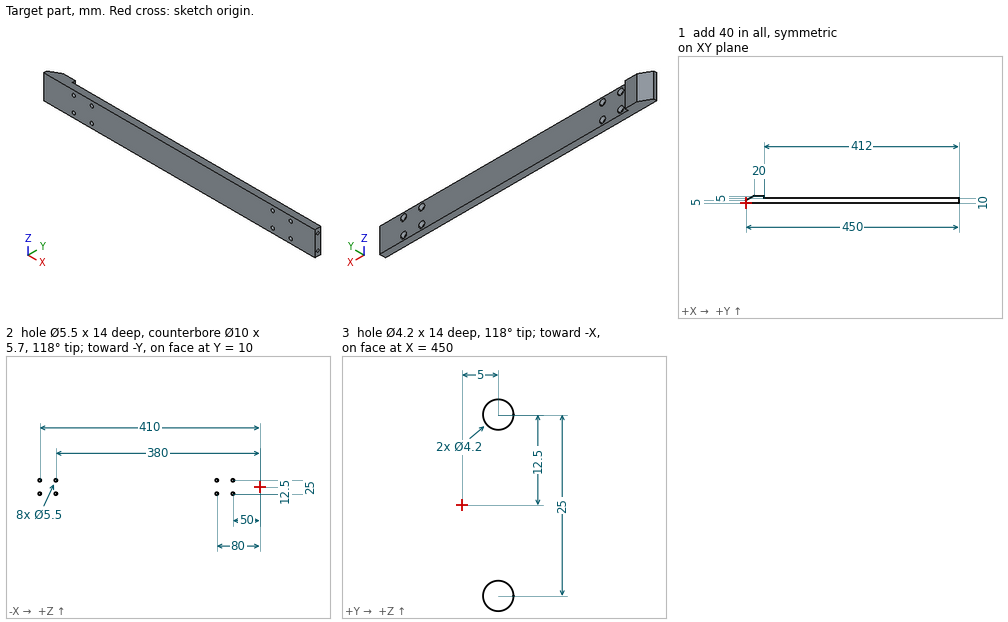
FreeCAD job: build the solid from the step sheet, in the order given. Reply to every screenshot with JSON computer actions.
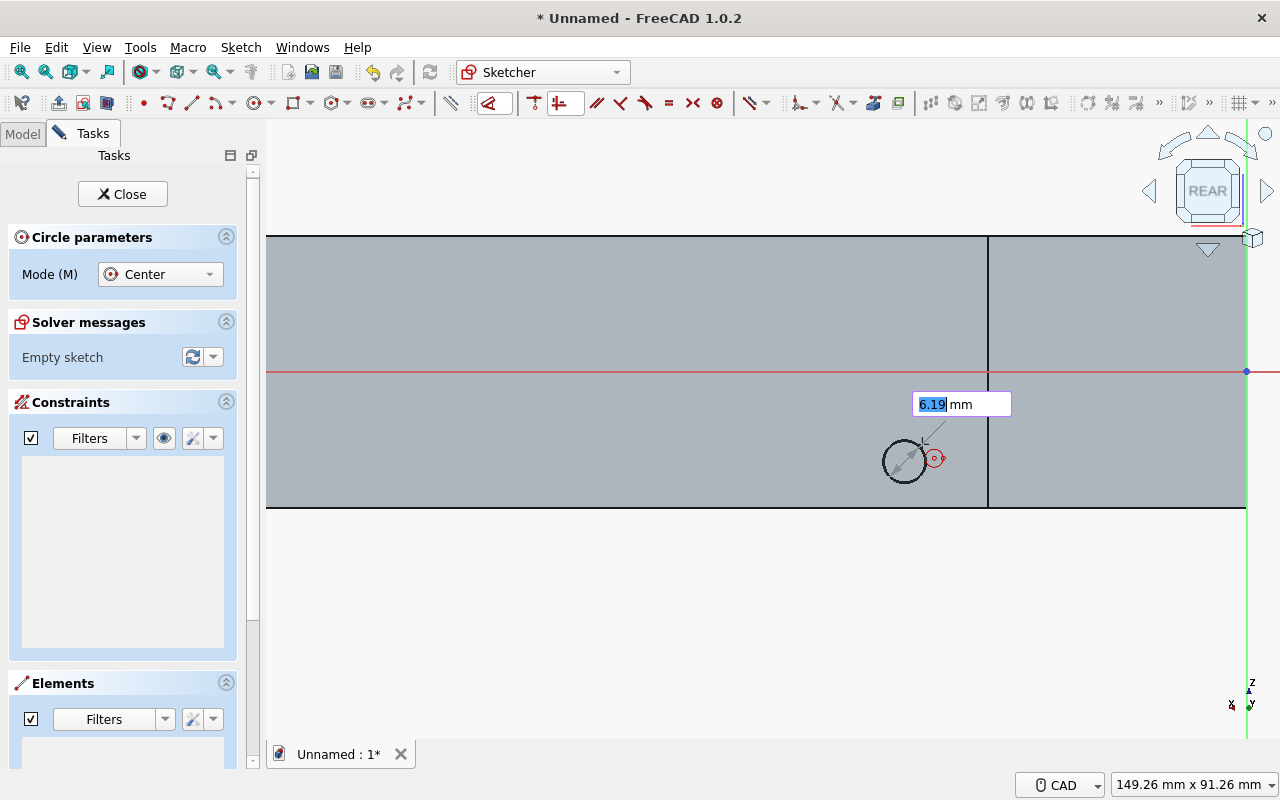
{"action": "left_click", "coordinate": [920, 443]}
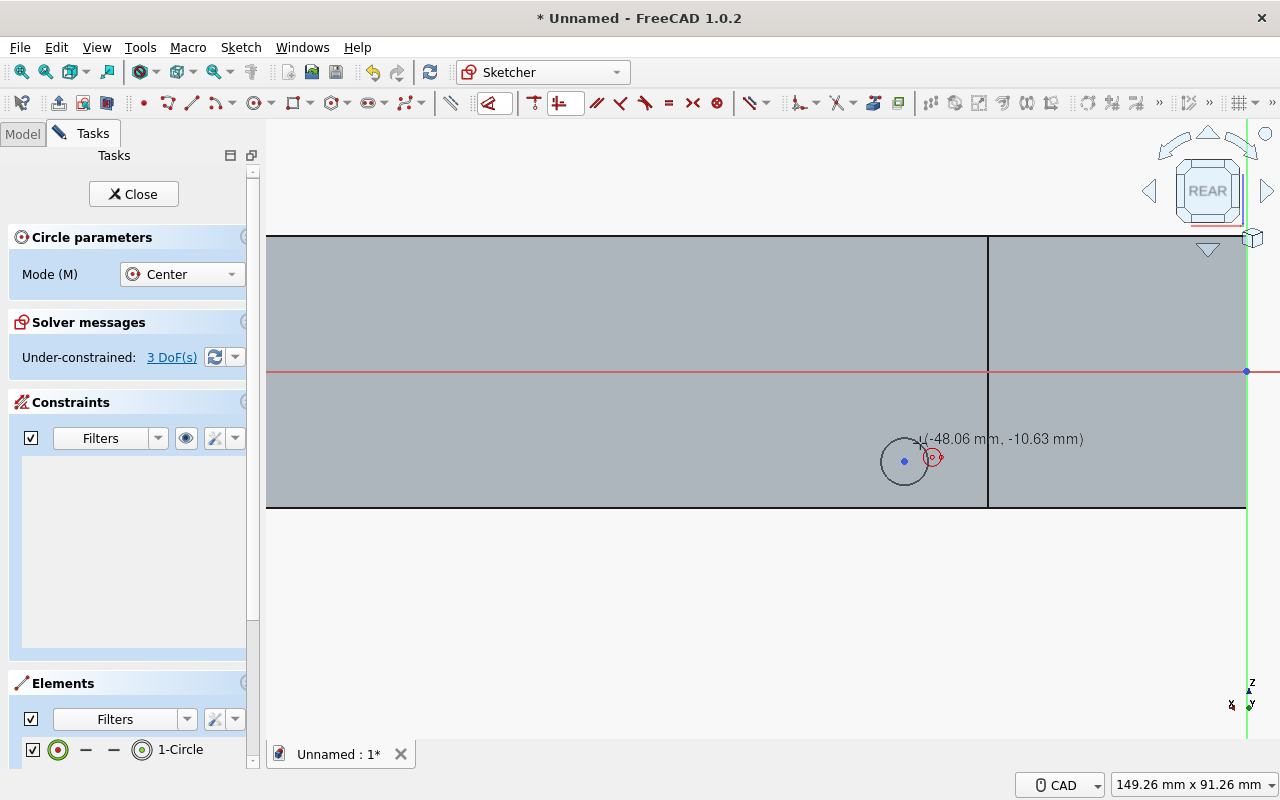
{"action": "scroll", "coordinate": [922, 443], "scroll_direction": "down", "scroll_amount": 8}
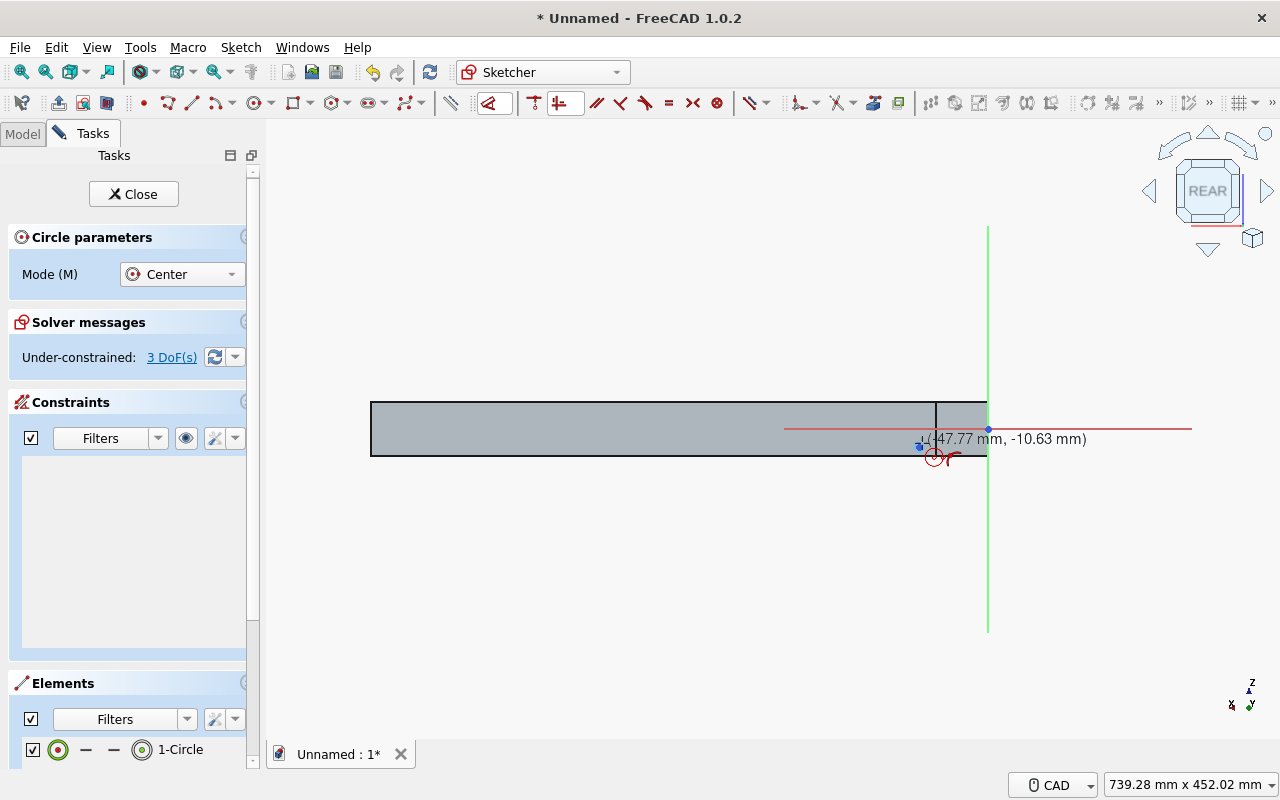
{"action": "left_click", "coordinate": [878, 446]}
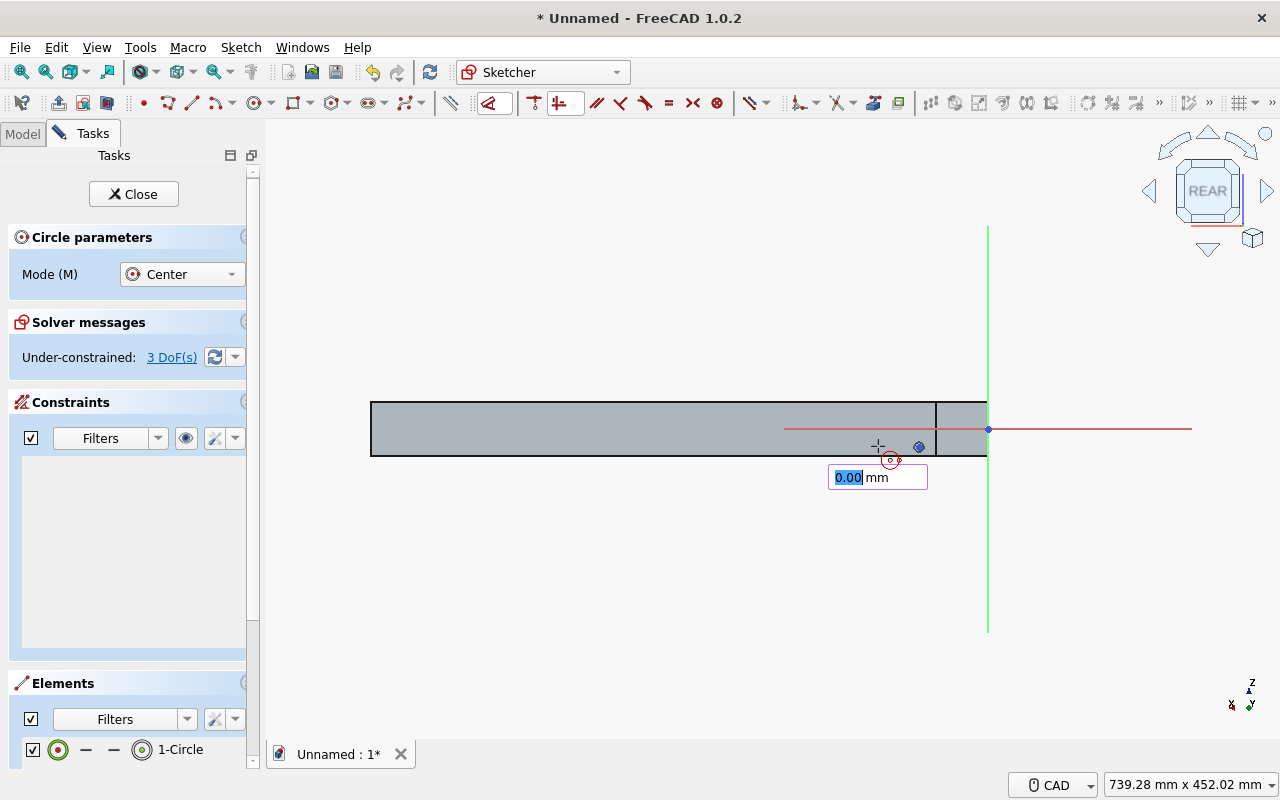
{"action": "scroll", "coordinate": [881, 444], "scroll_direction": "up", "scroll_amount": 8}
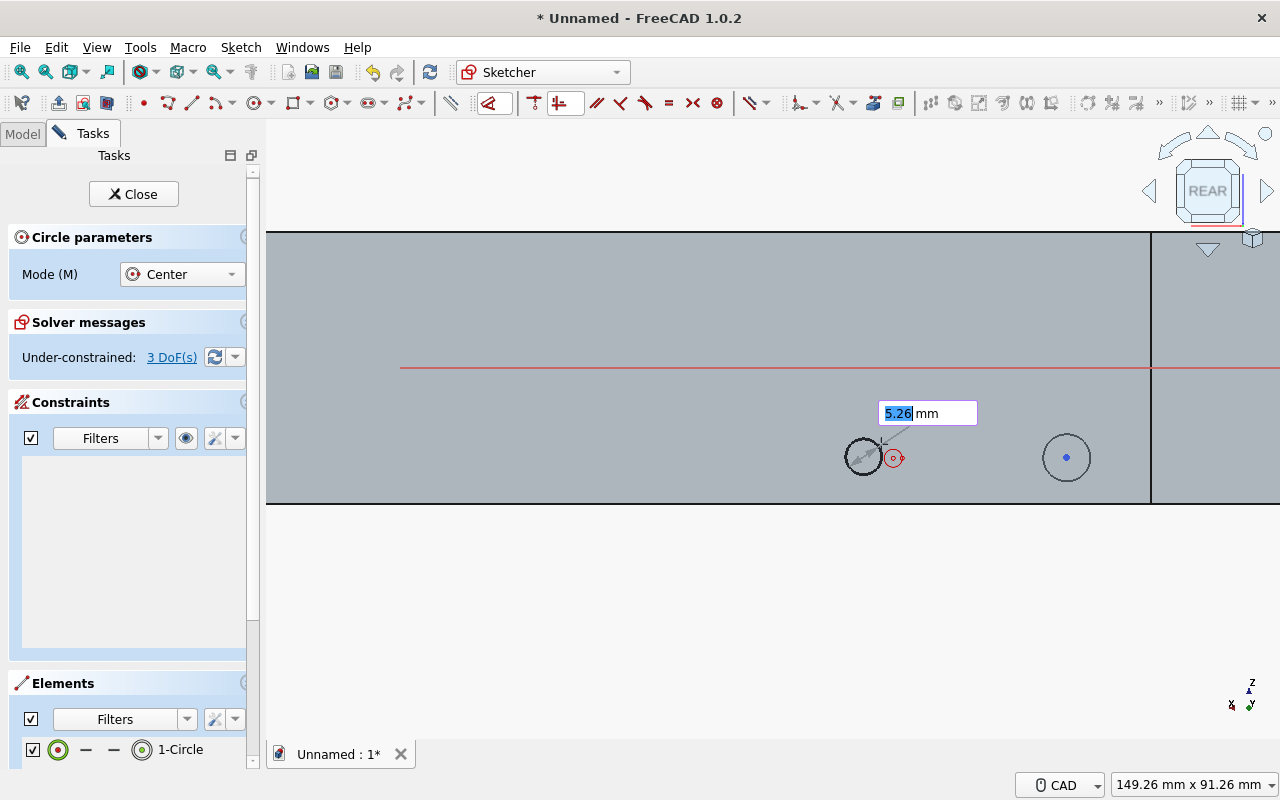
{"action": "left_click", "coordinate": [878, 440]}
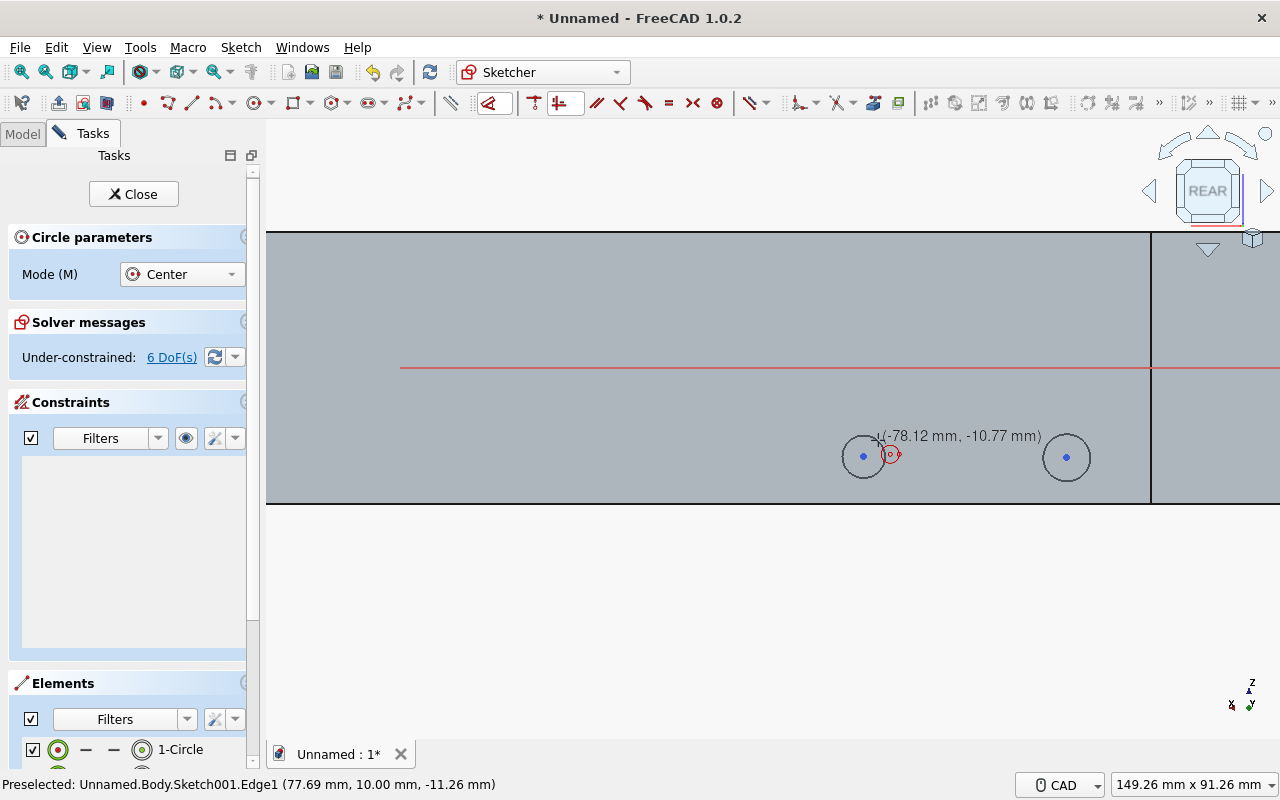
{"action": "scroll", "coordinate": [881, 444], "scroll_direction": "down", "scroll_amount": 8}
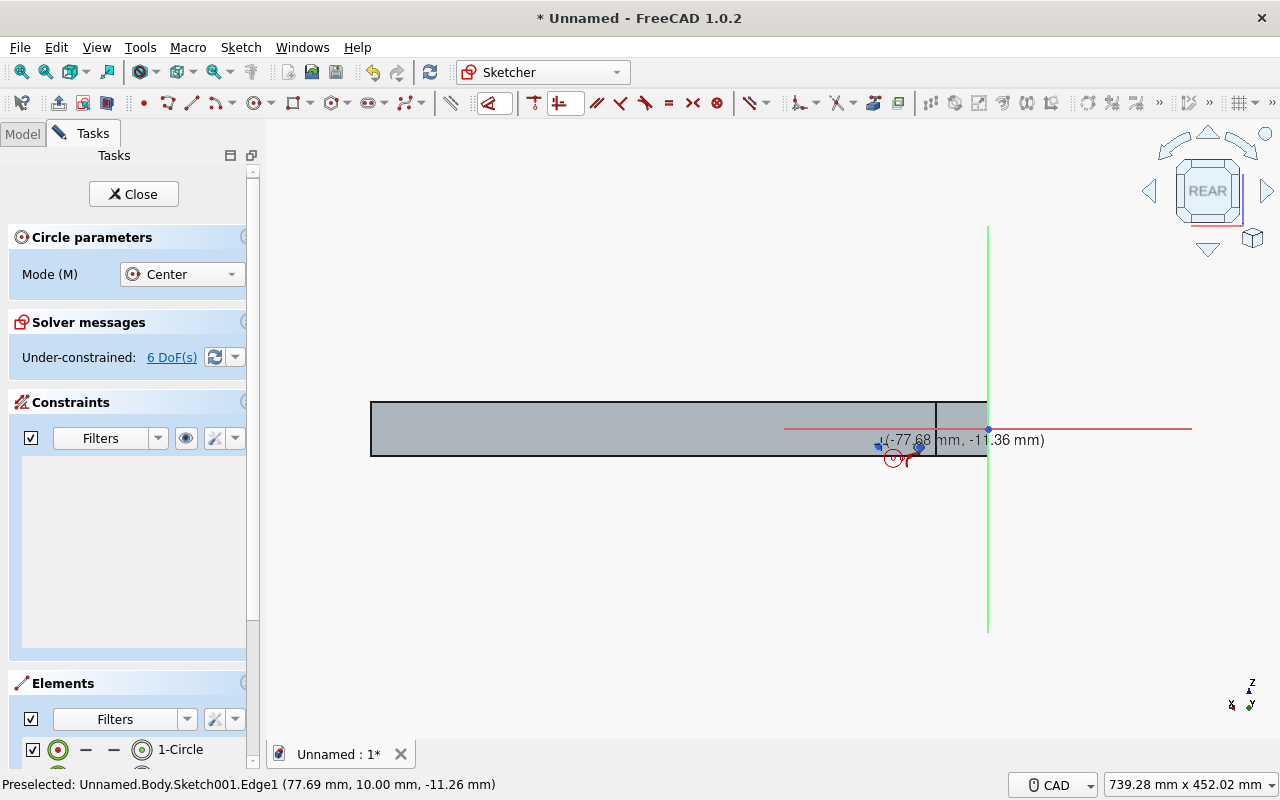
{"action": "left_click", "coordinate": [919, 412]}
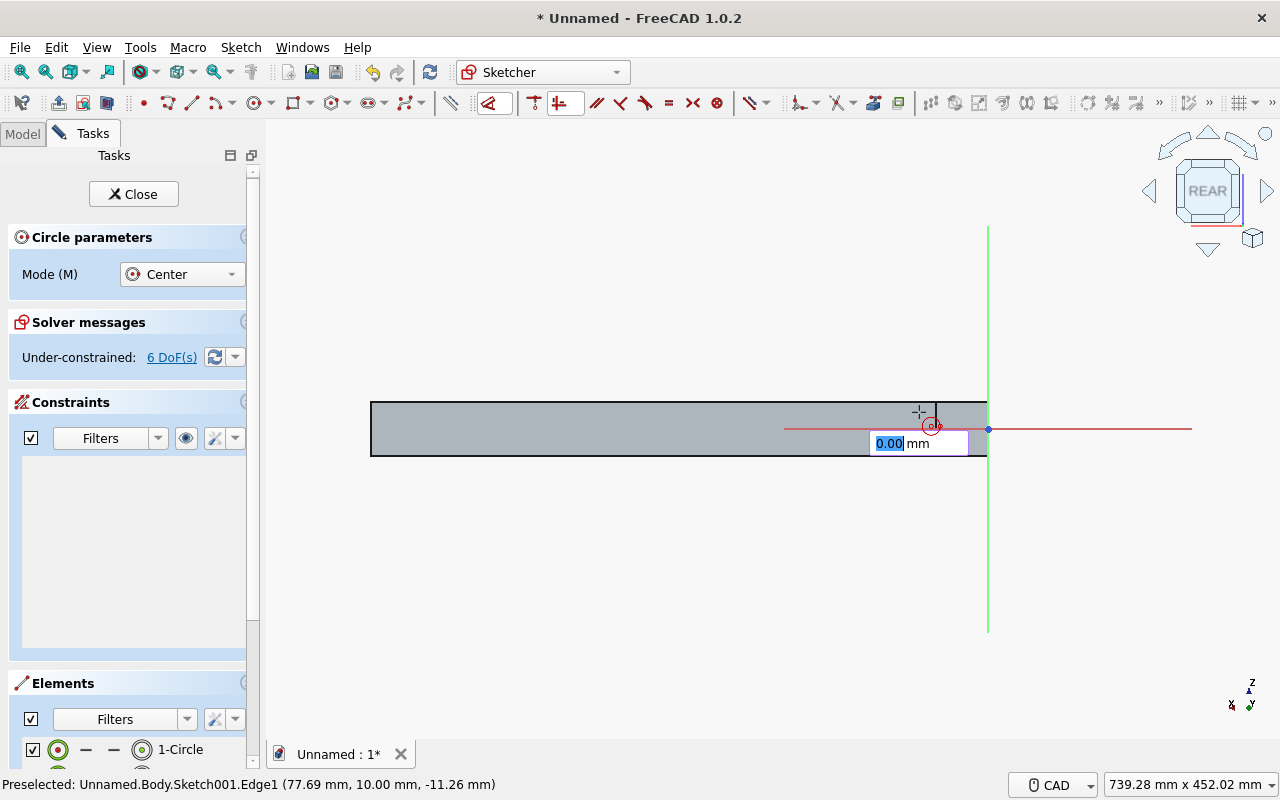
{"action": "scroll", "coordinate": [922, 409], "scroll_direction": "up", "scroll_amount": 8}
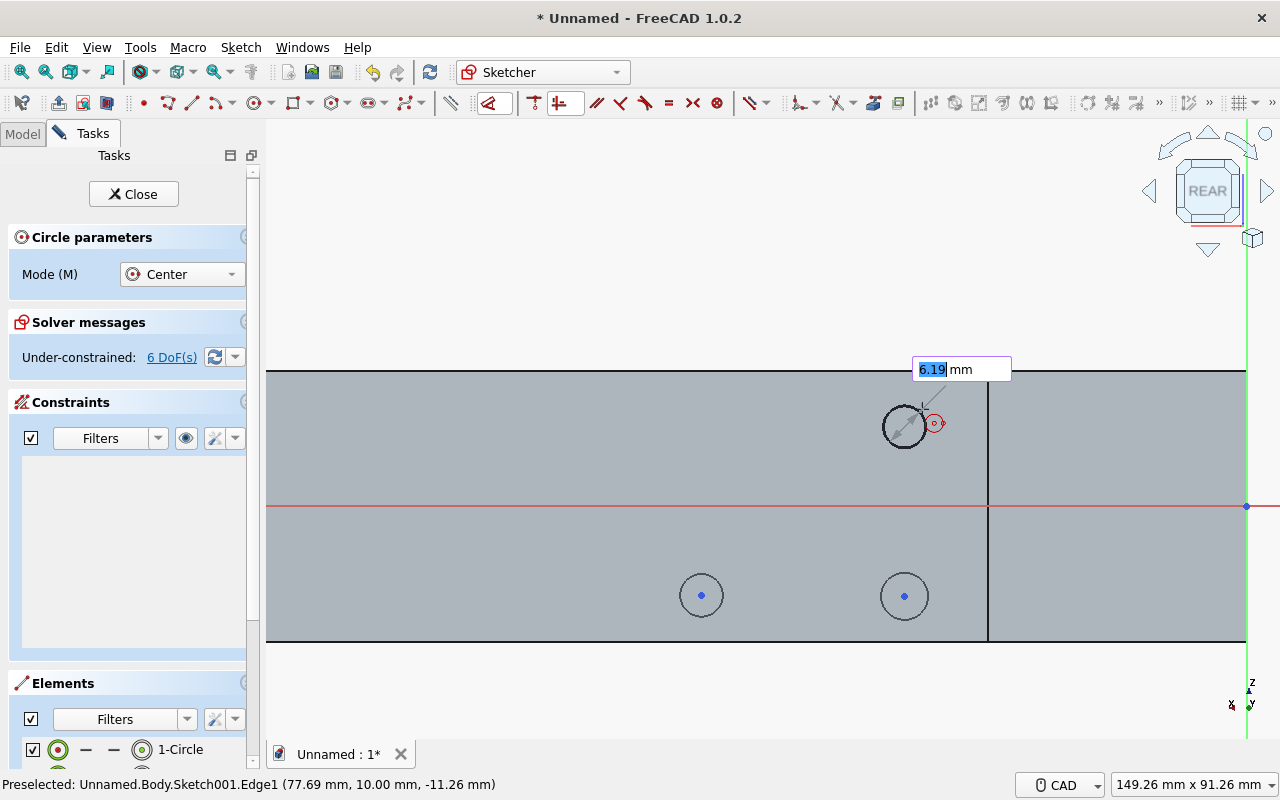
{"action": "left_click", "coordinate": [920, 408]}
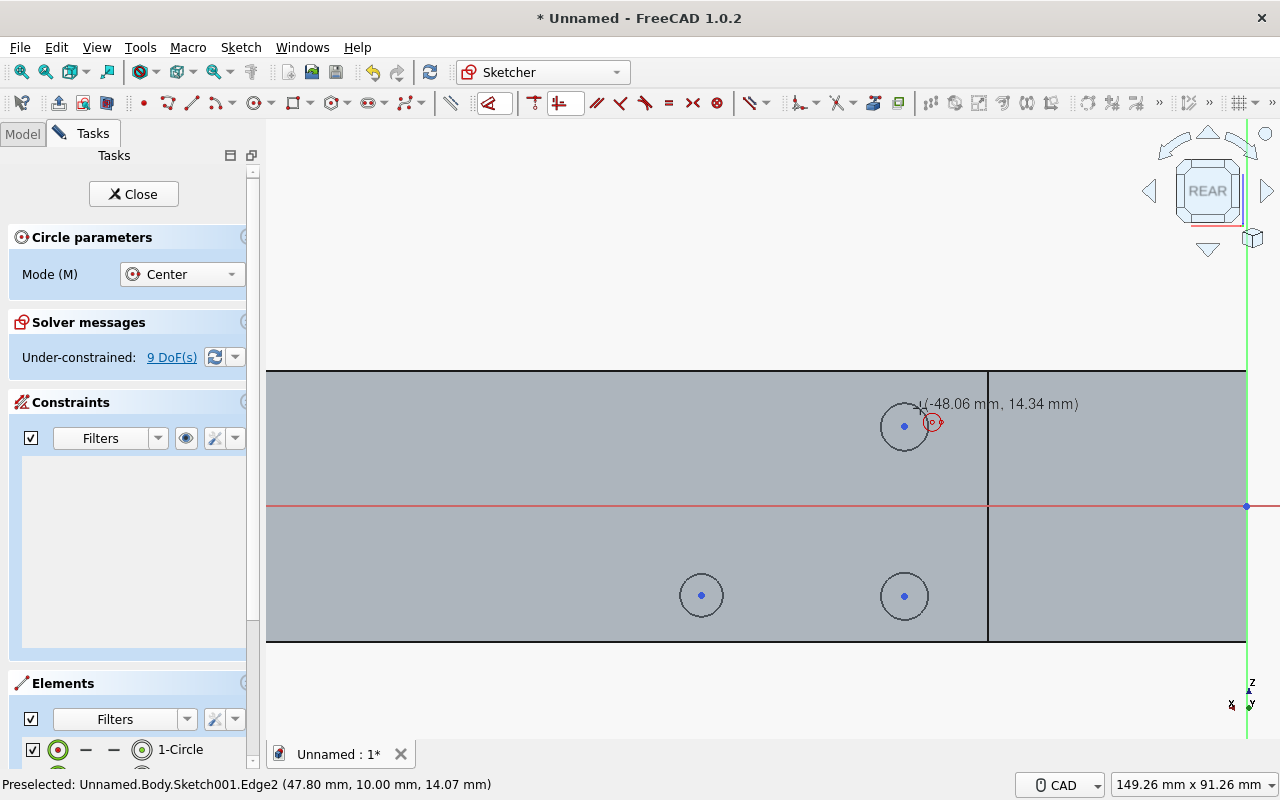
{"action": "scroll", "coordinate": [922, 409], "scroll_direction": "down", "scroll_amount": 8}